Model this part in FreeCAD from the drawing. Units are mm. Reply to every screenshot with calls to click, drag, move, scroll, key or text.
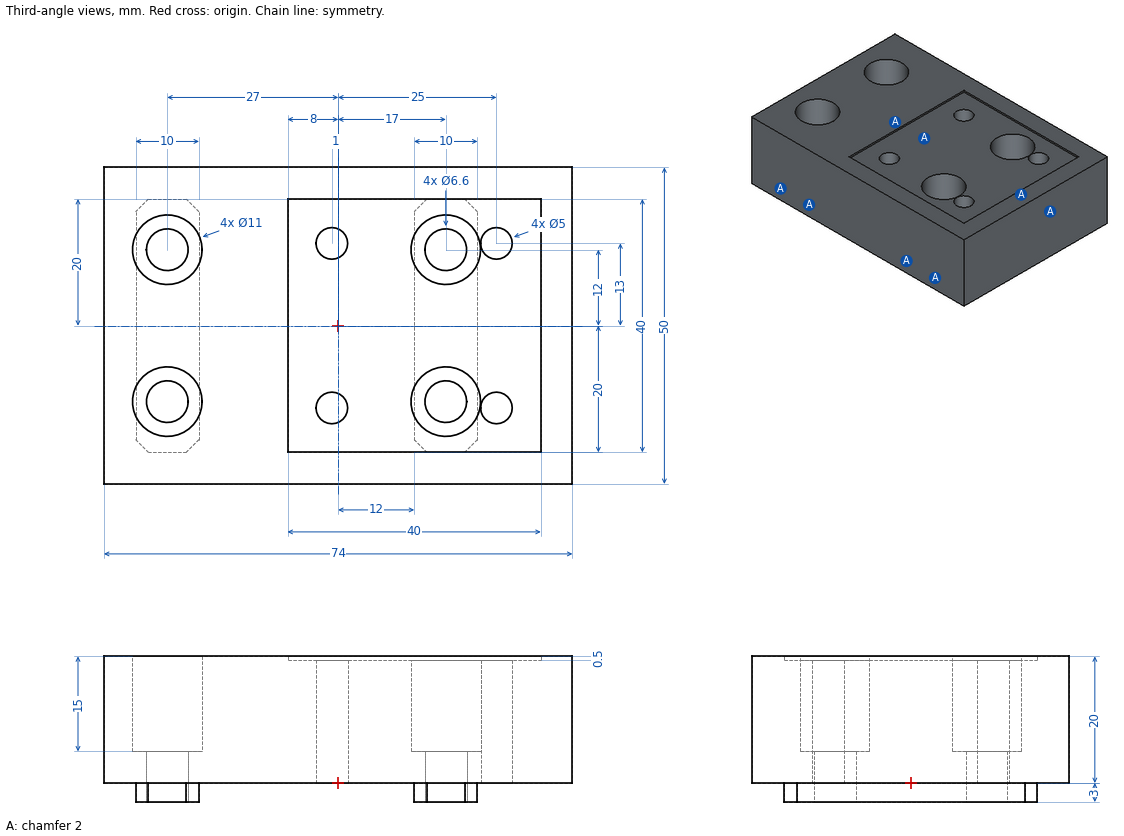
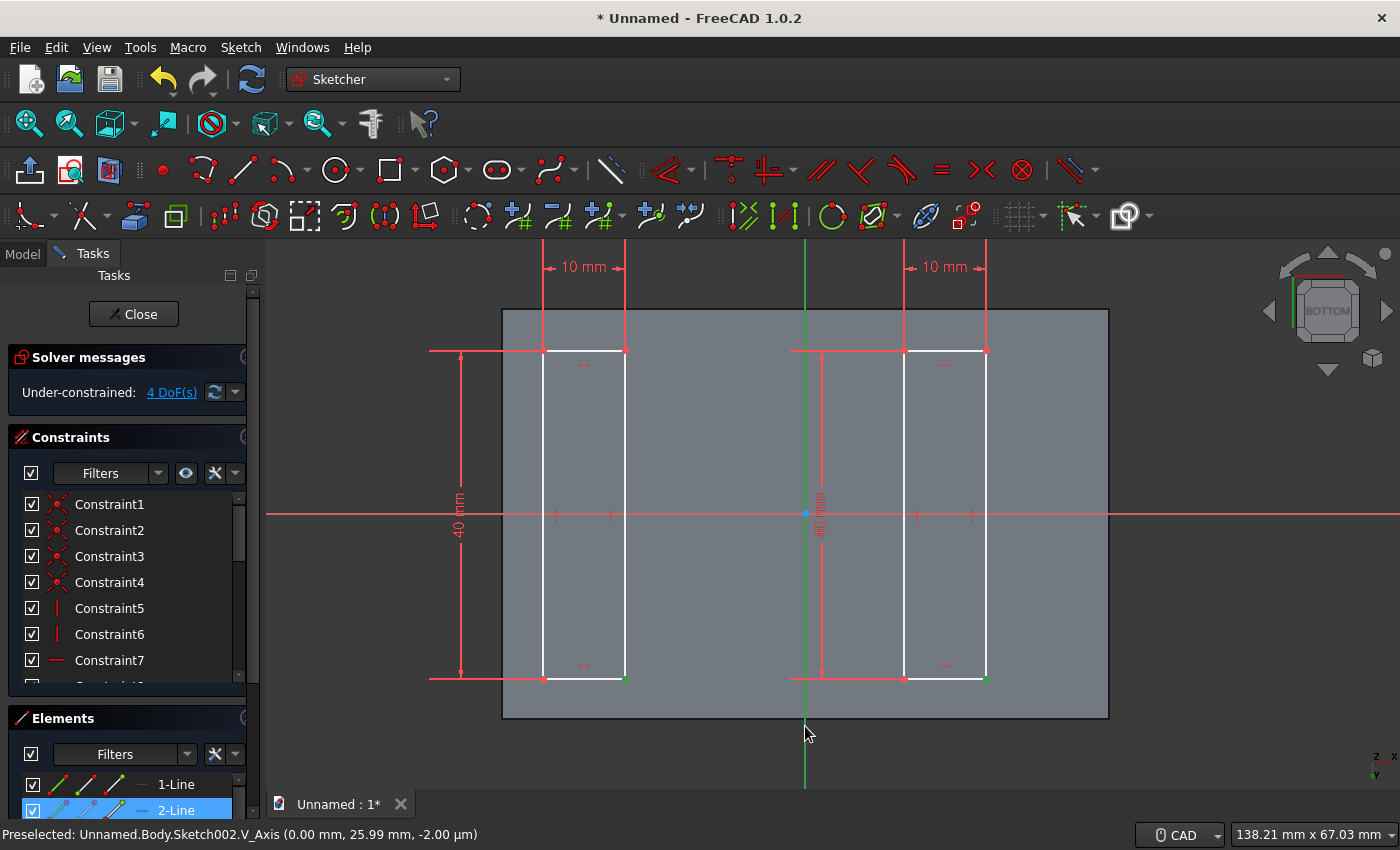
click(982, 170)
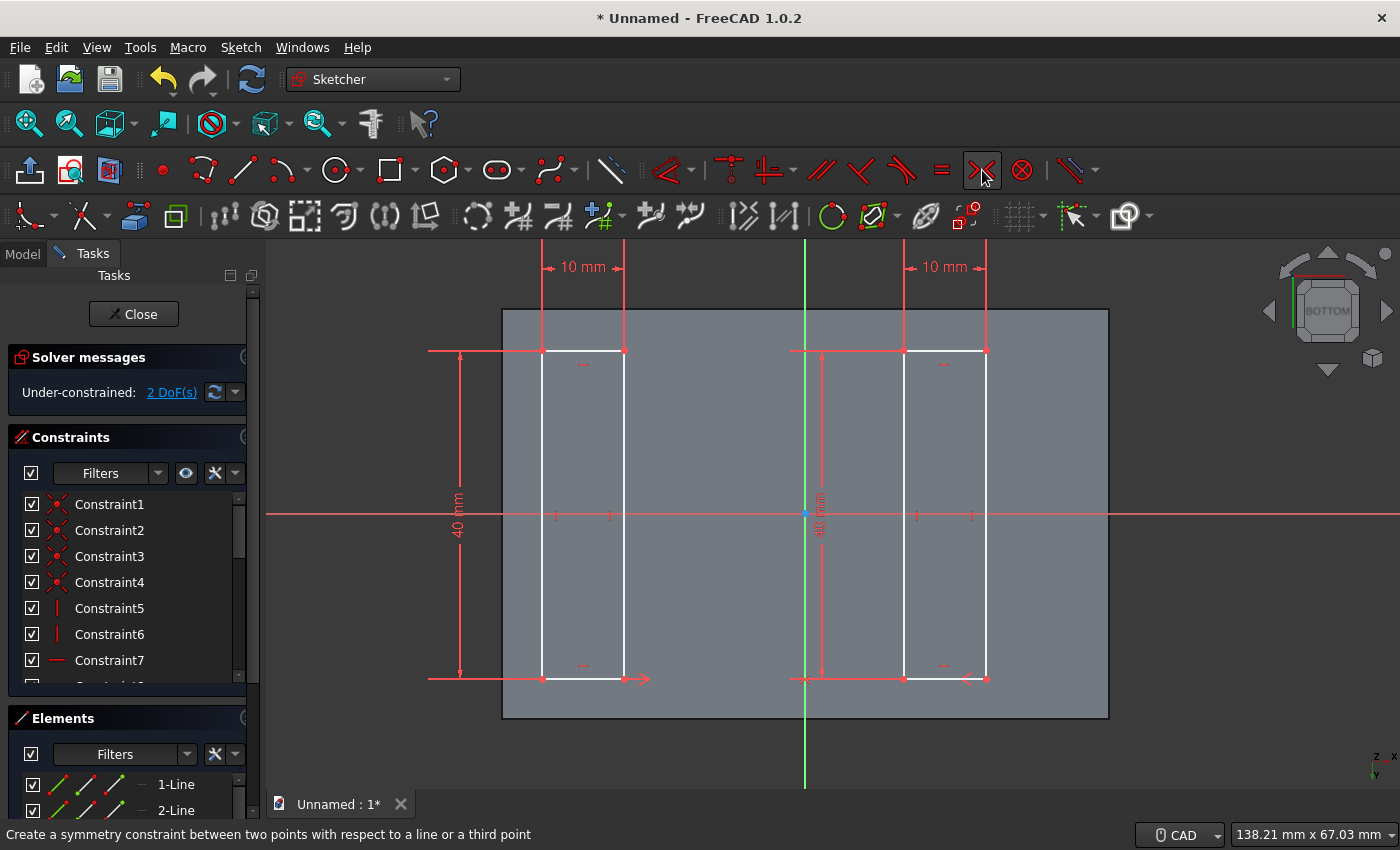
click(666, 170)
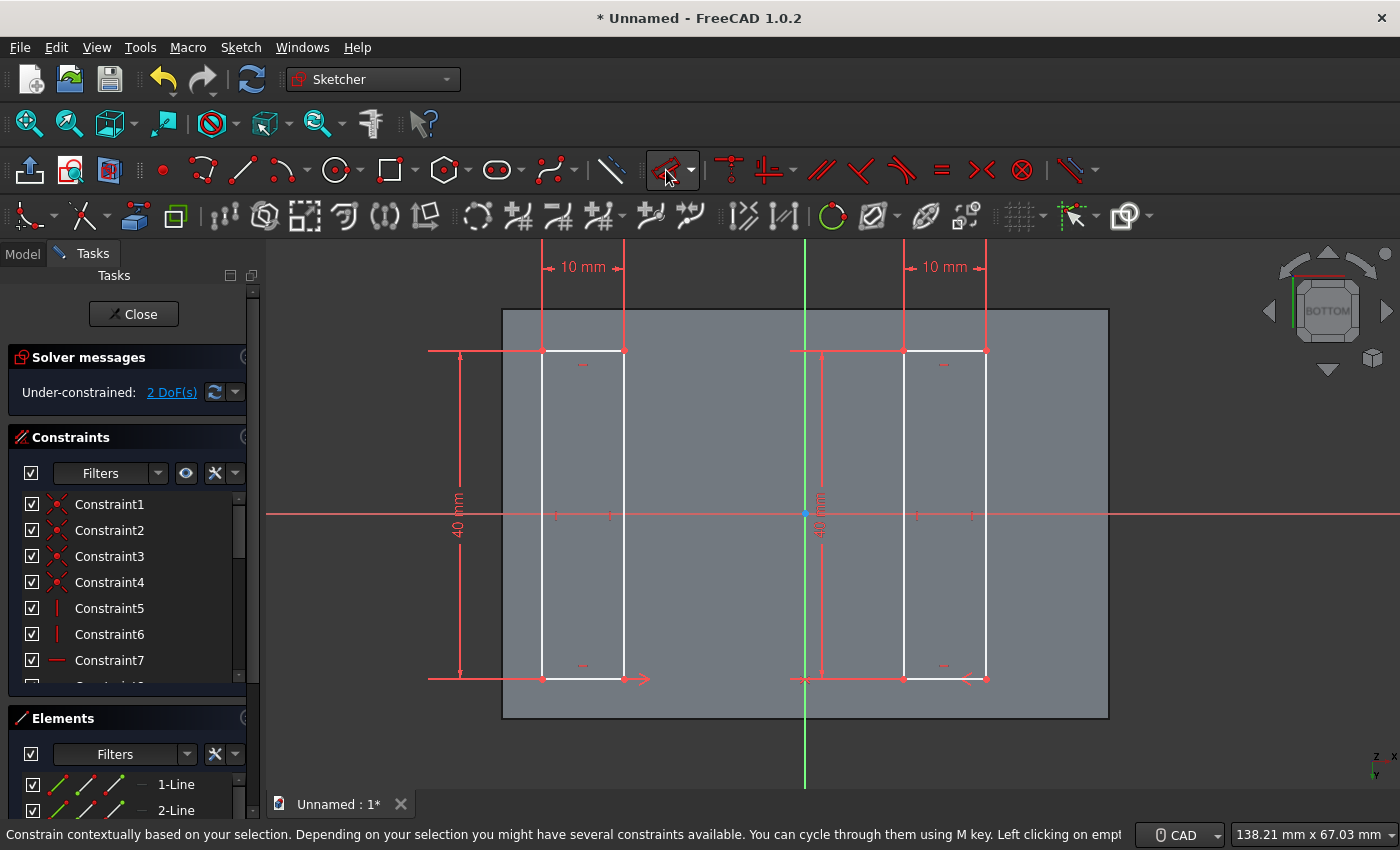
click(904, 351)
click(855, 317)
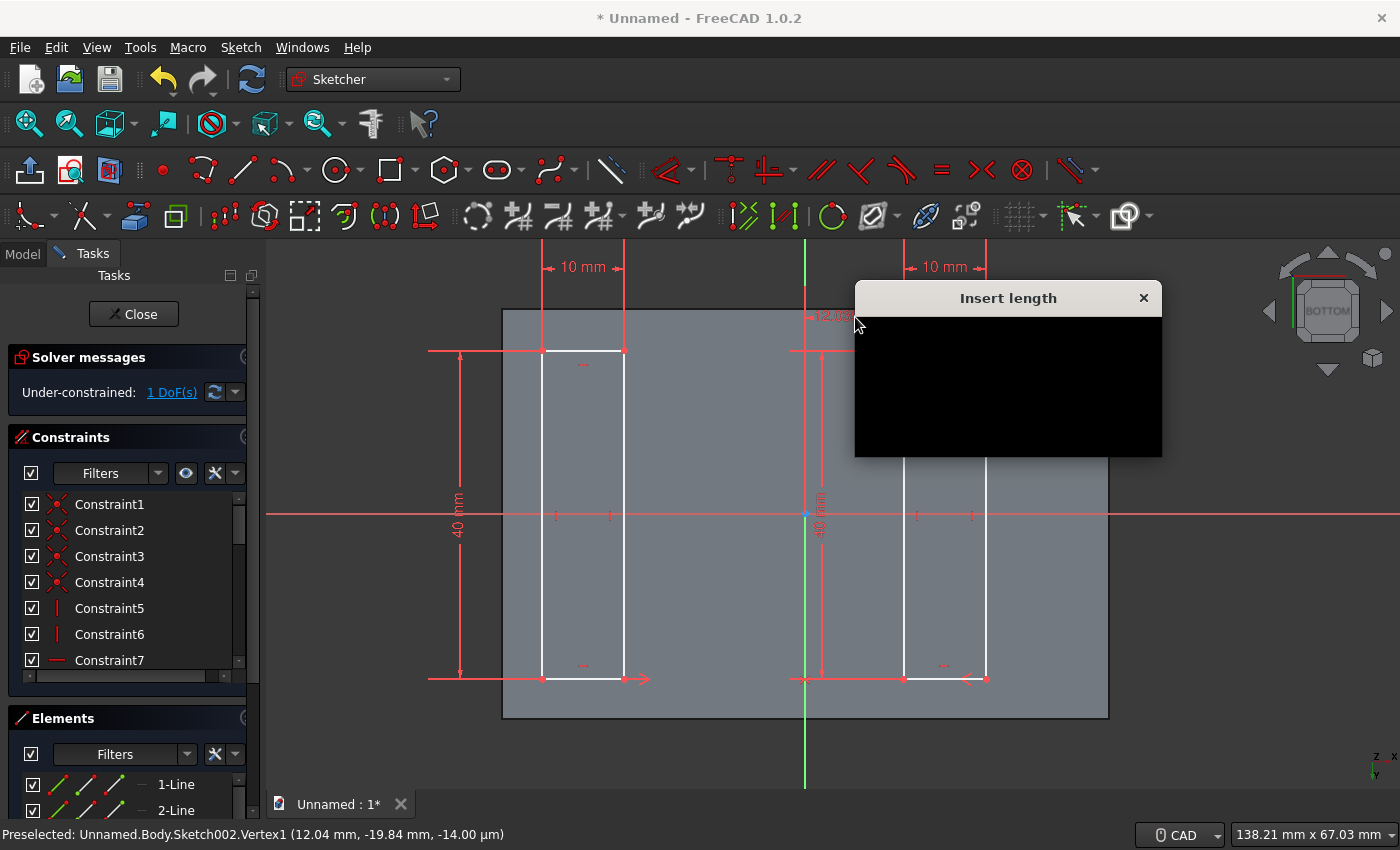
text(12)
key(Return)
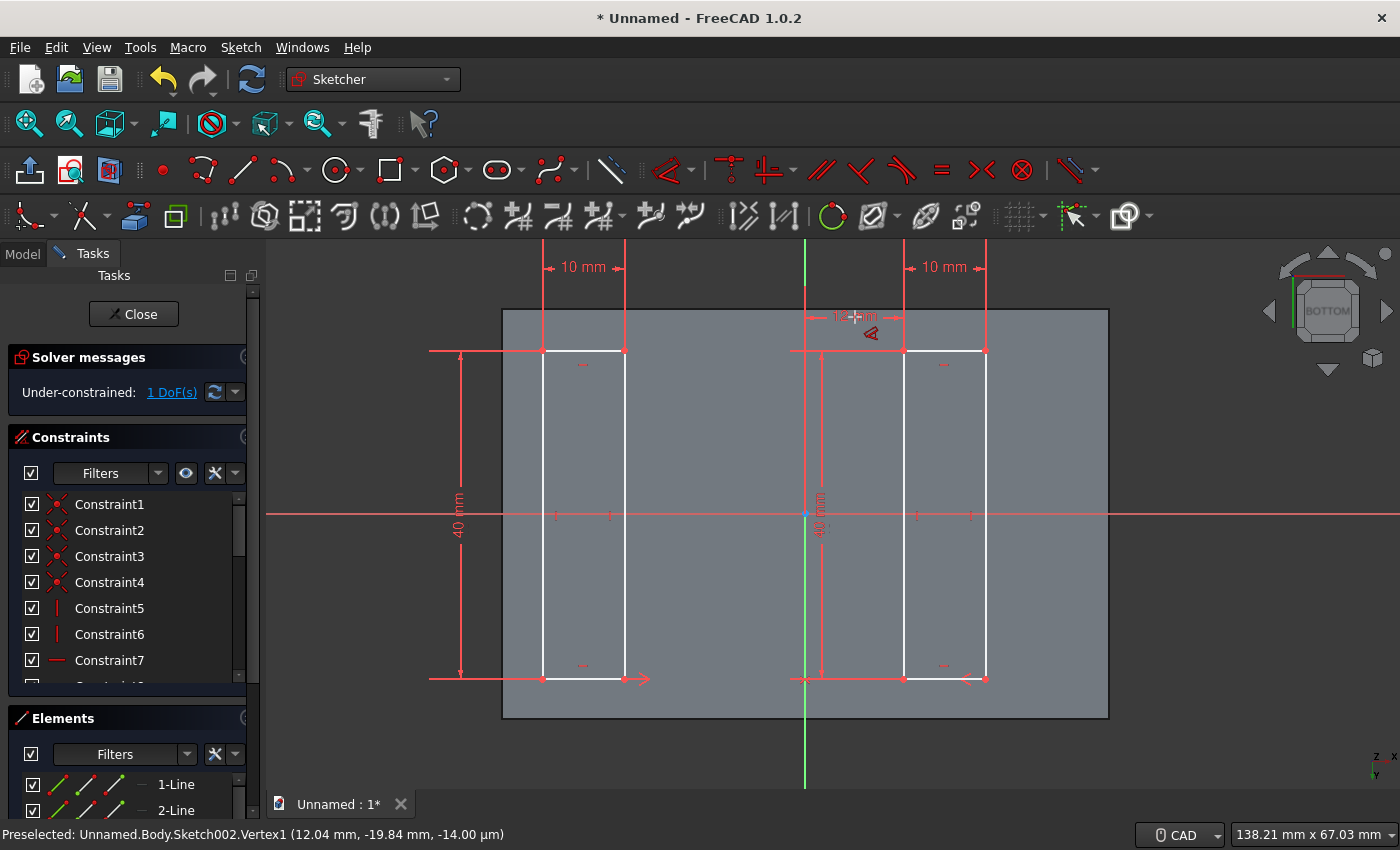
click(904, 351)
click(938, 432)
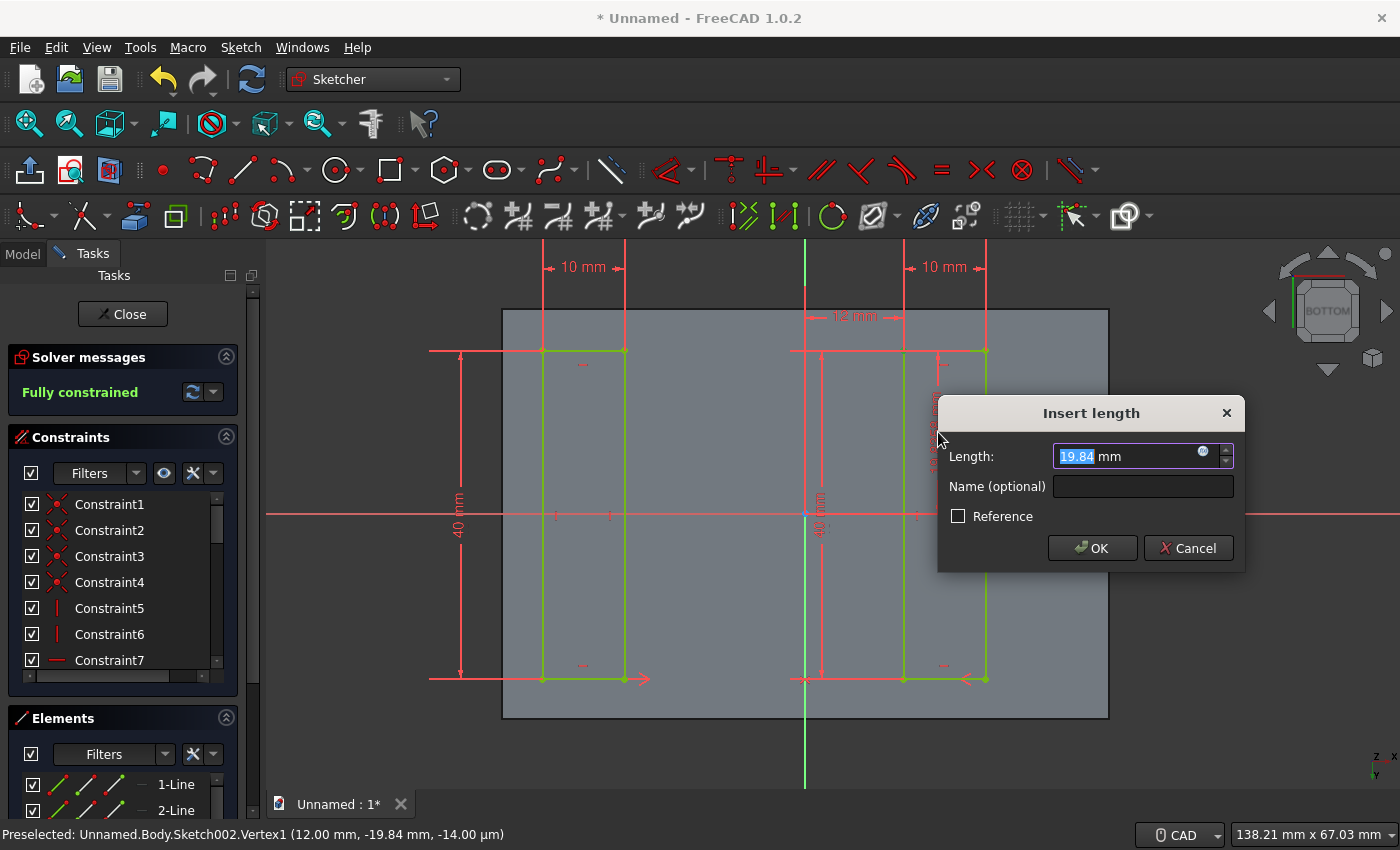
text(20)
key(Return)
key(Escape)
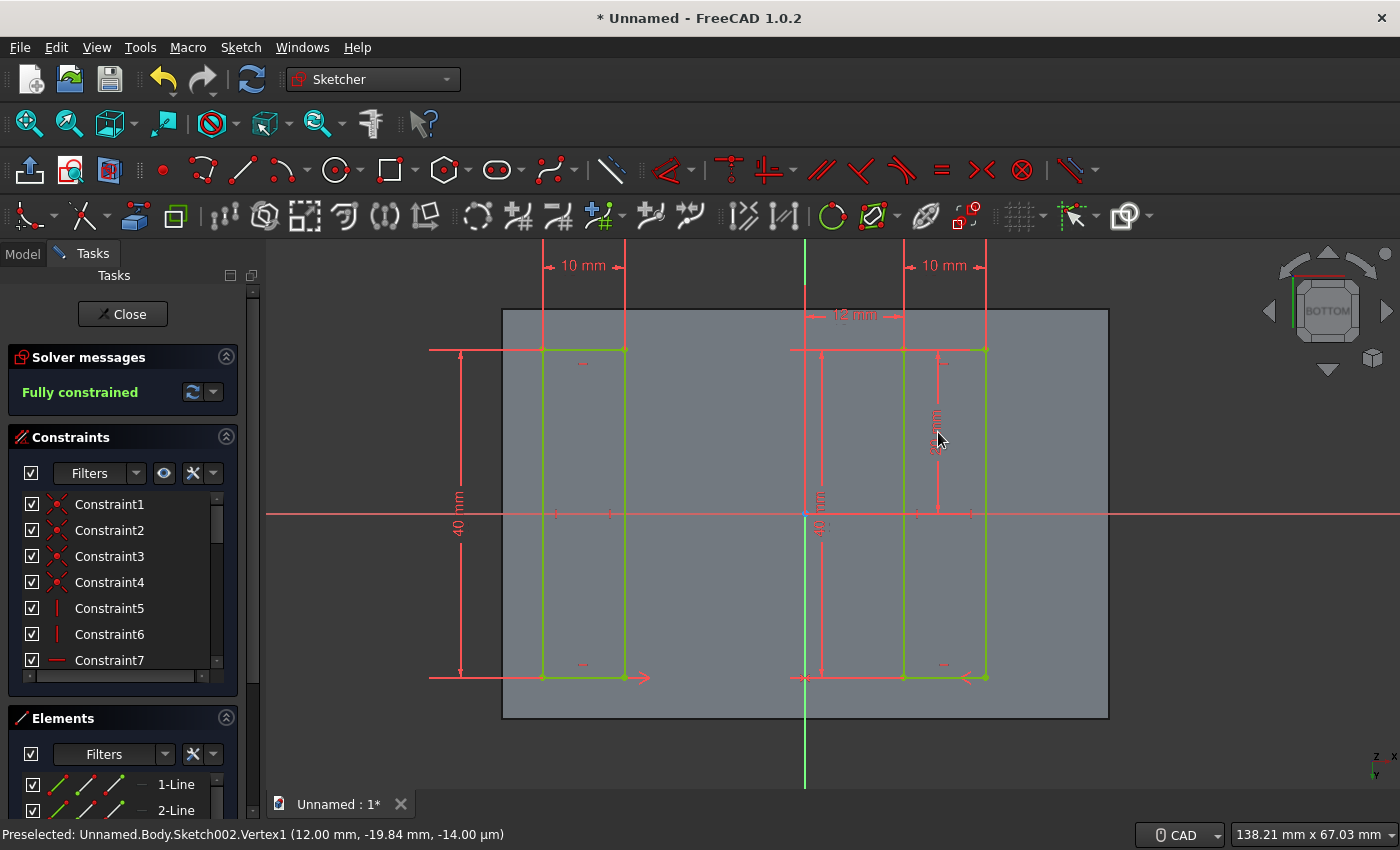
click(123, 314)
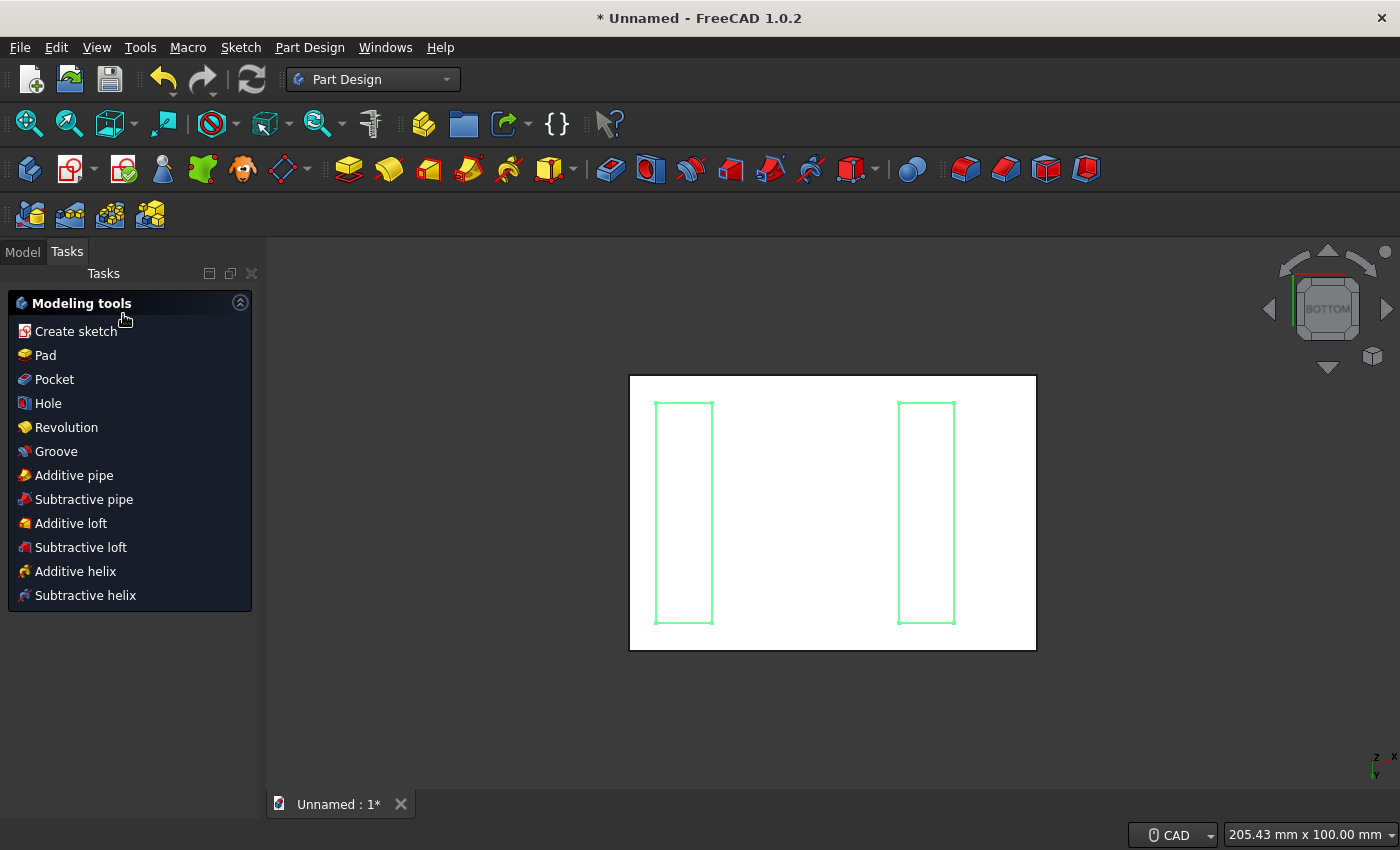
click(350, 170)